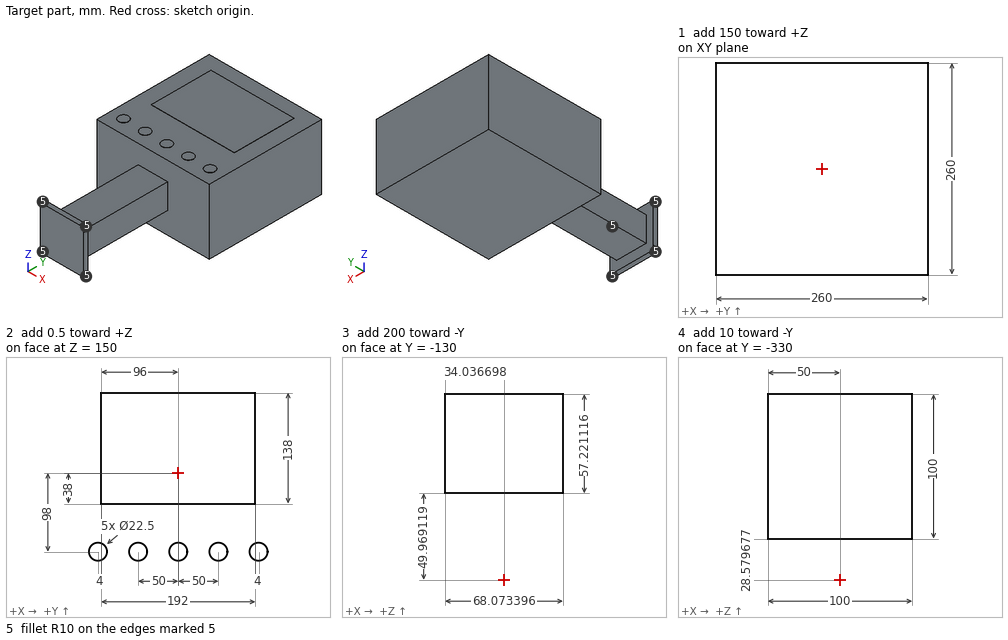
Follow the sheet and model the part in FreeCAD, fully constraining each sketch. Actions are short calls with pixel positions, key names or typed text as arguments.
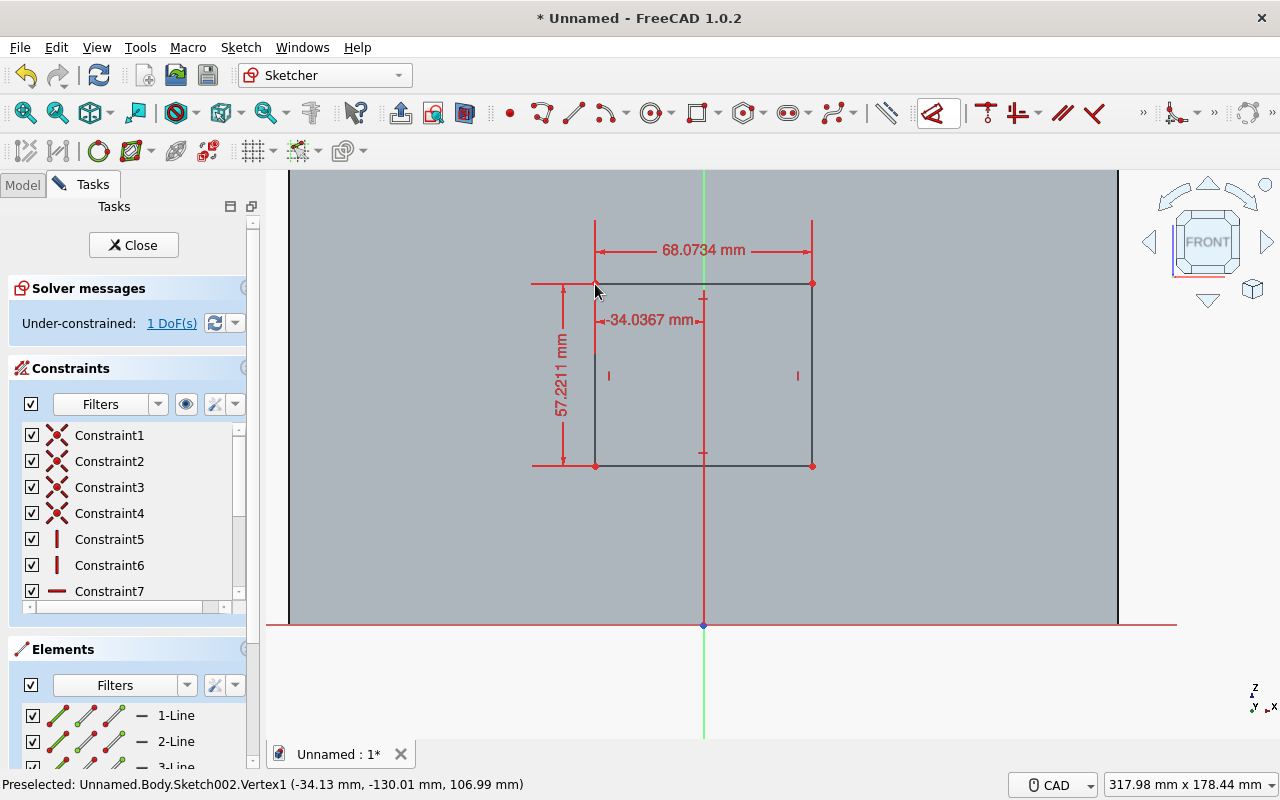
click(595, 466)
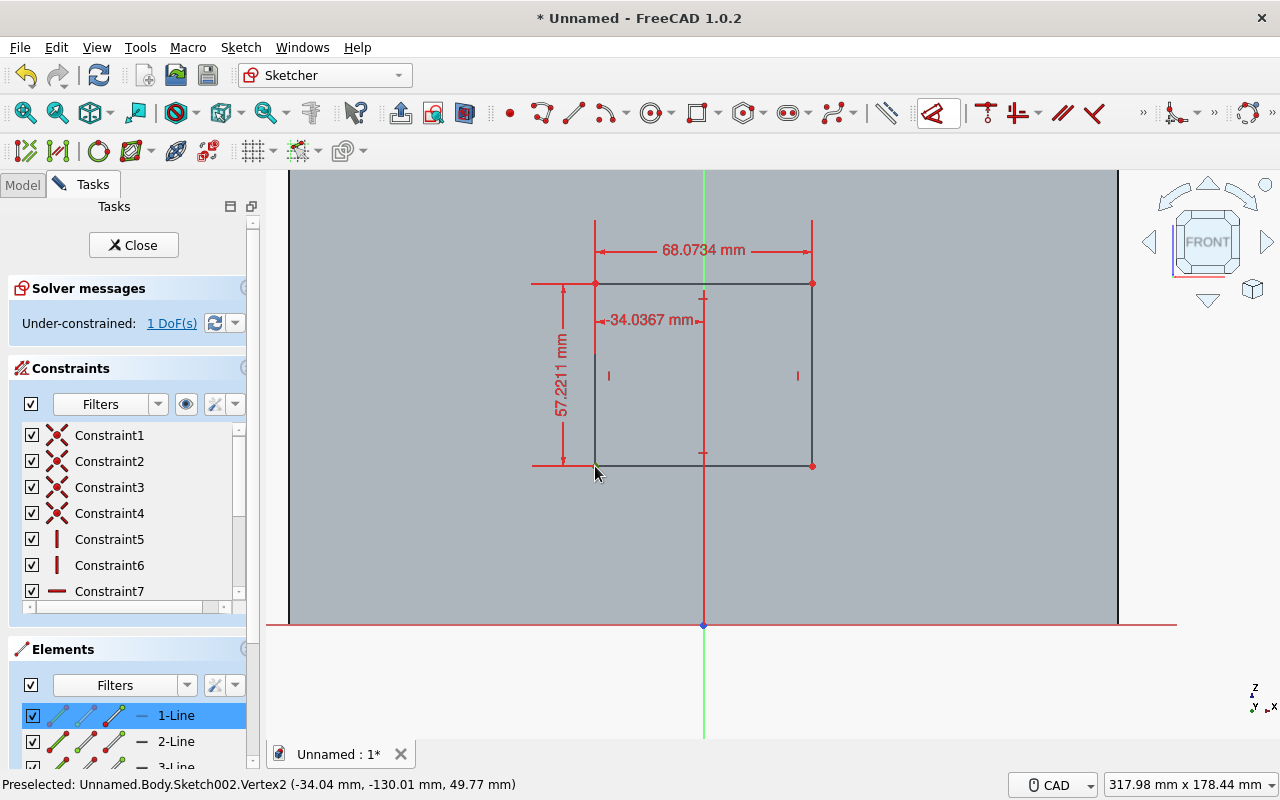
key(i)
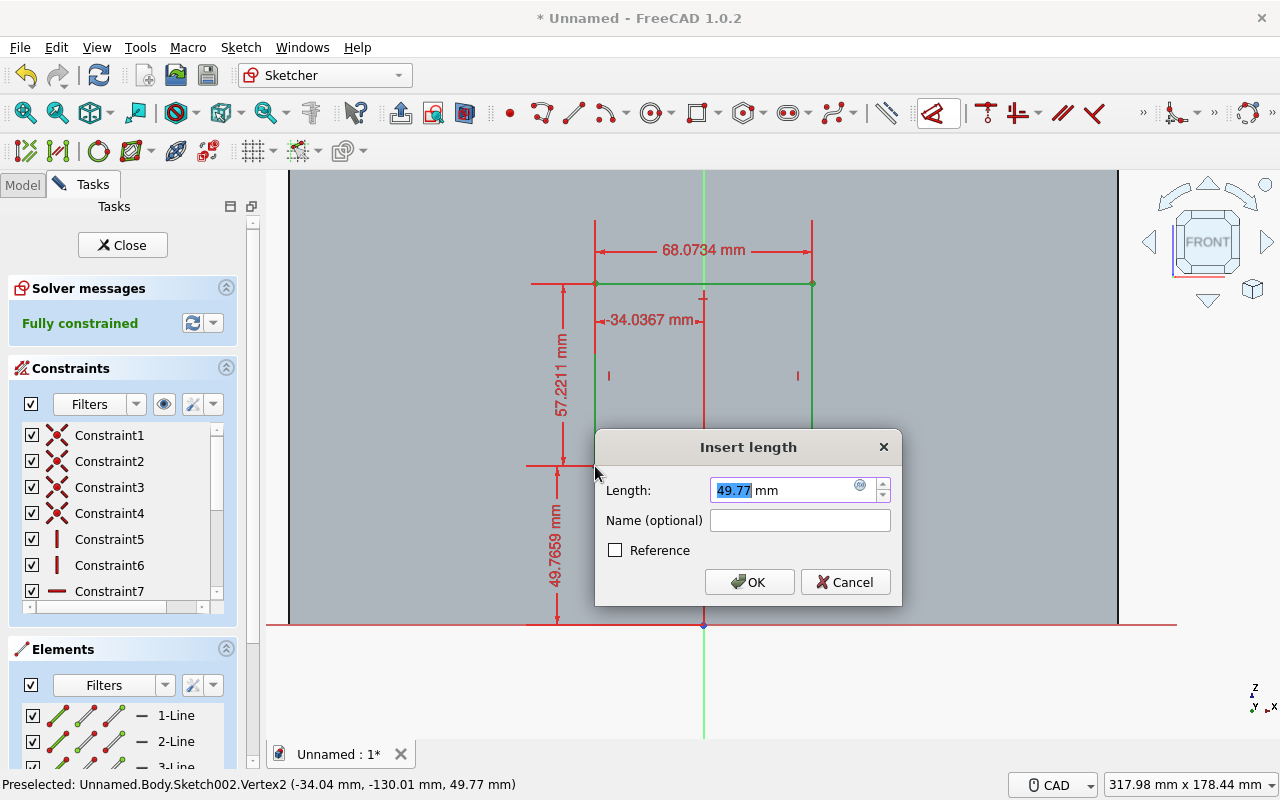
text(49.969119)
key(Return)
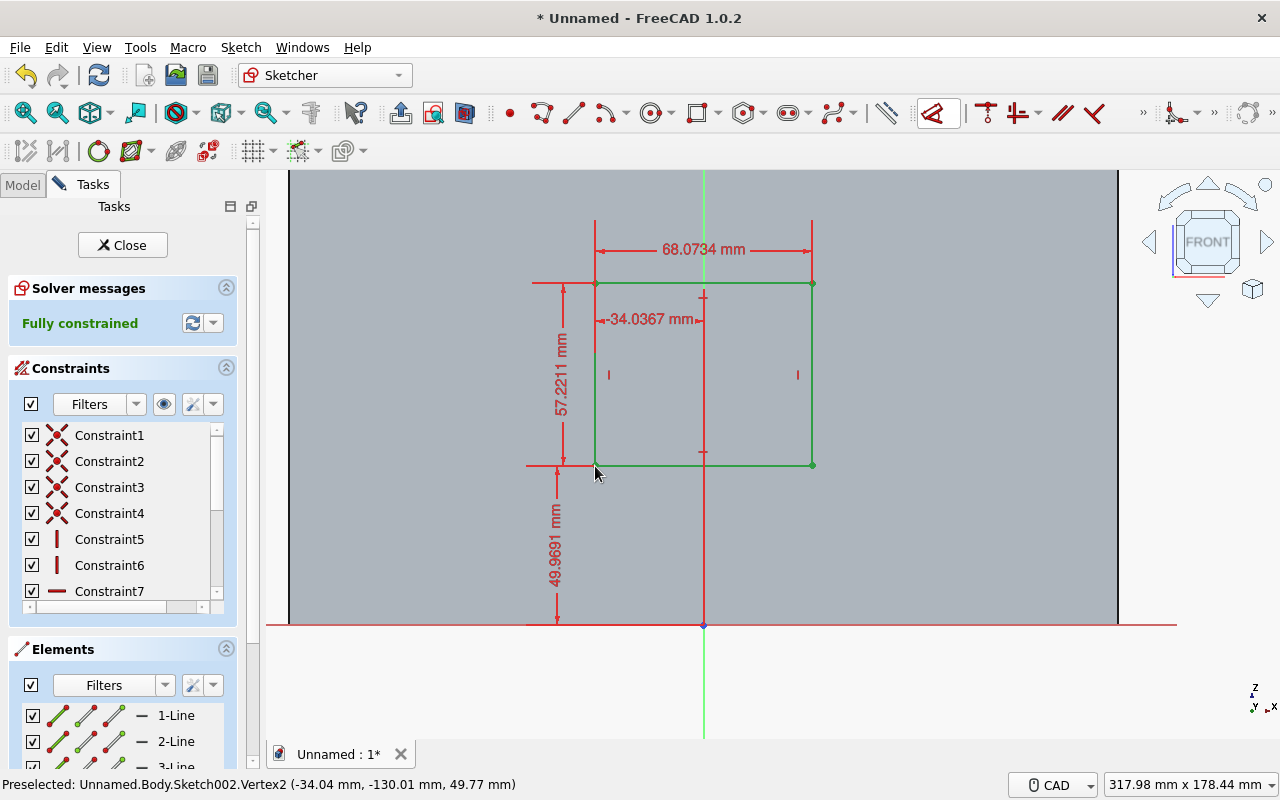
click(123, 245)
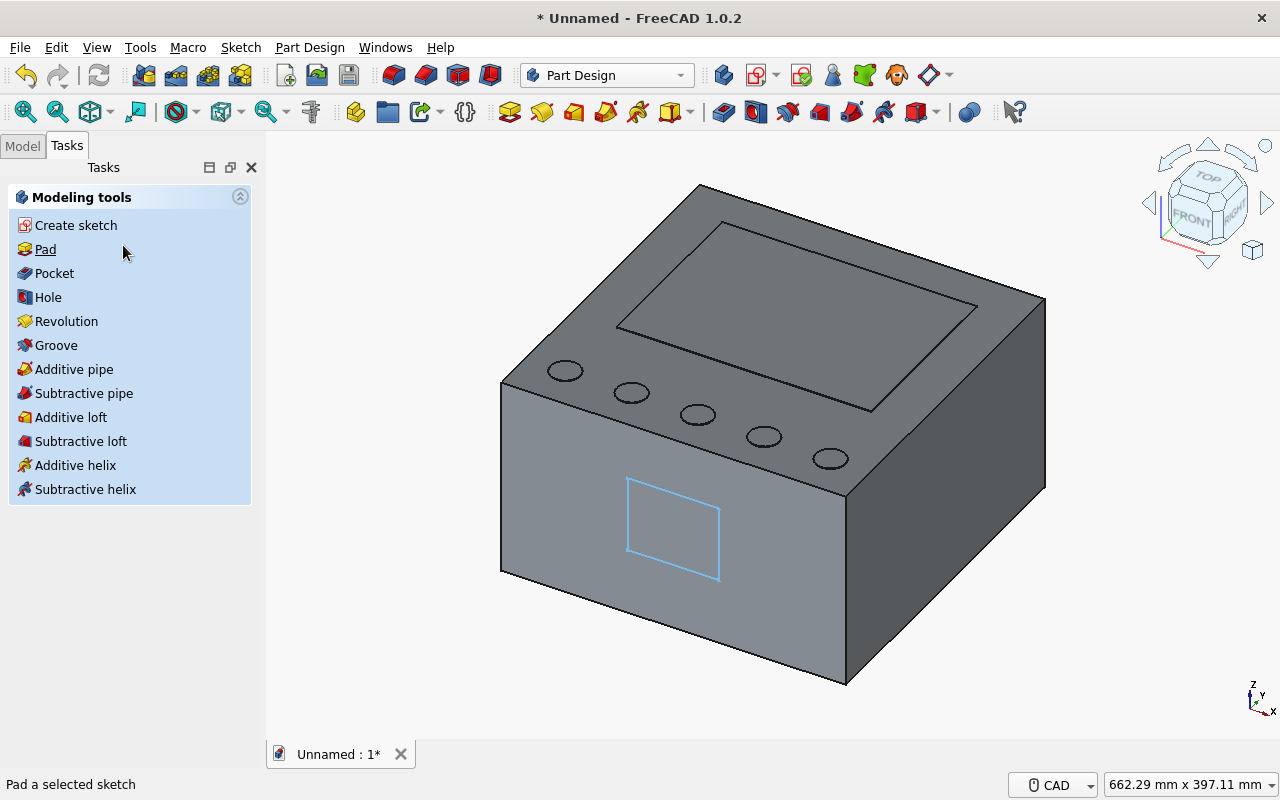
click(510, 112)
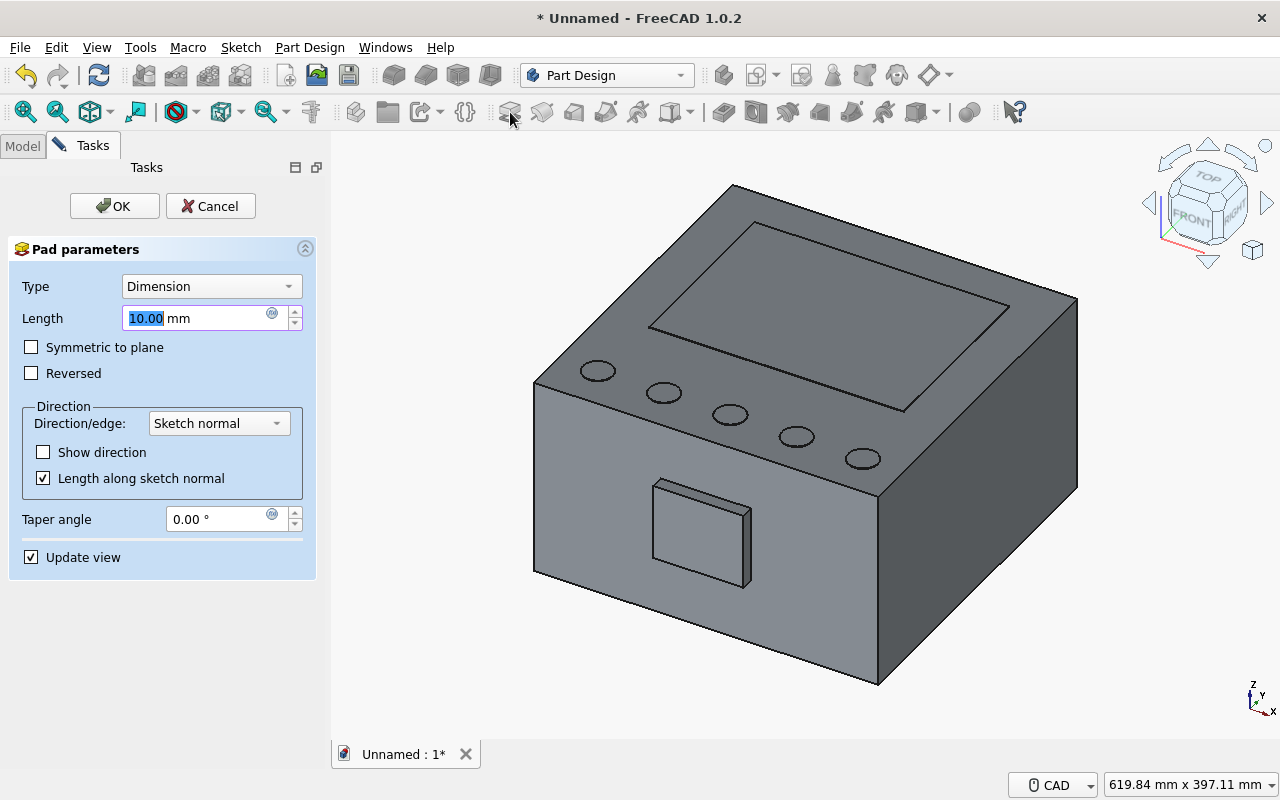
text(200)
key(Tab)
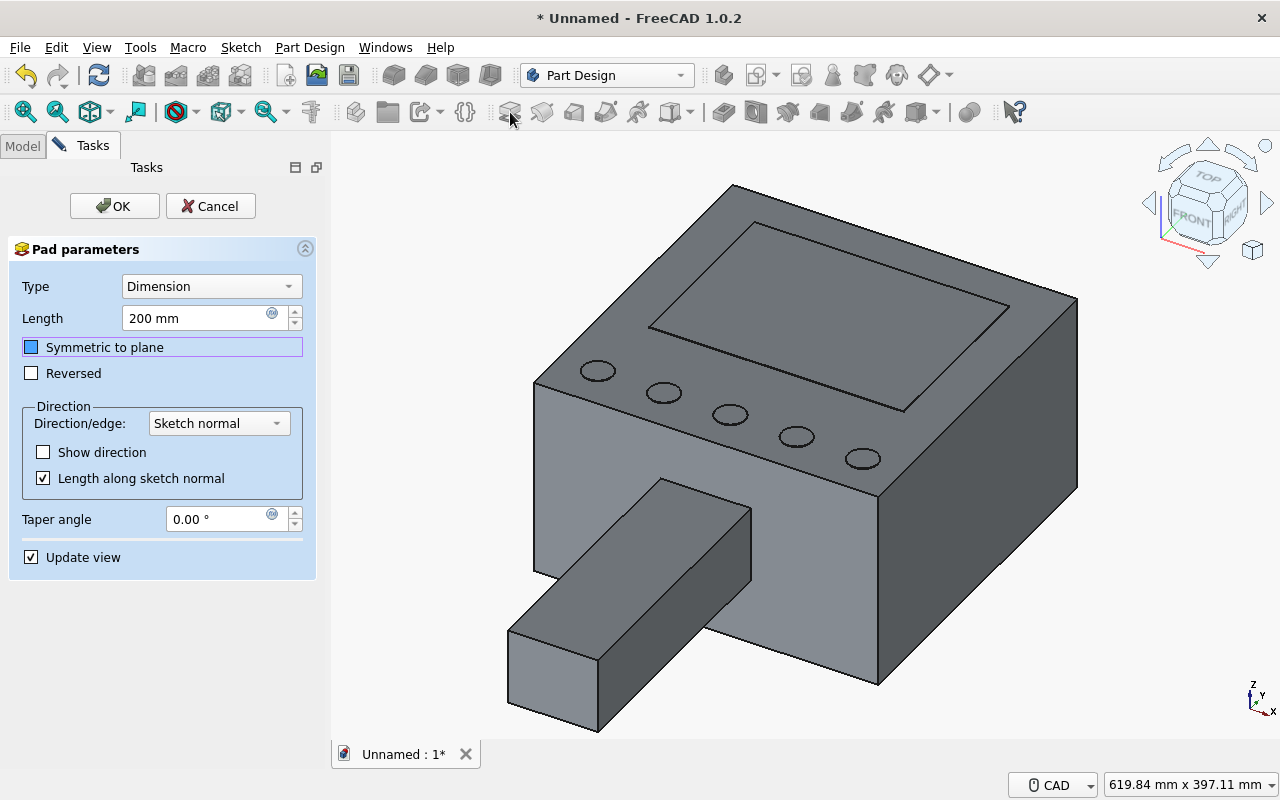
click(115, 206)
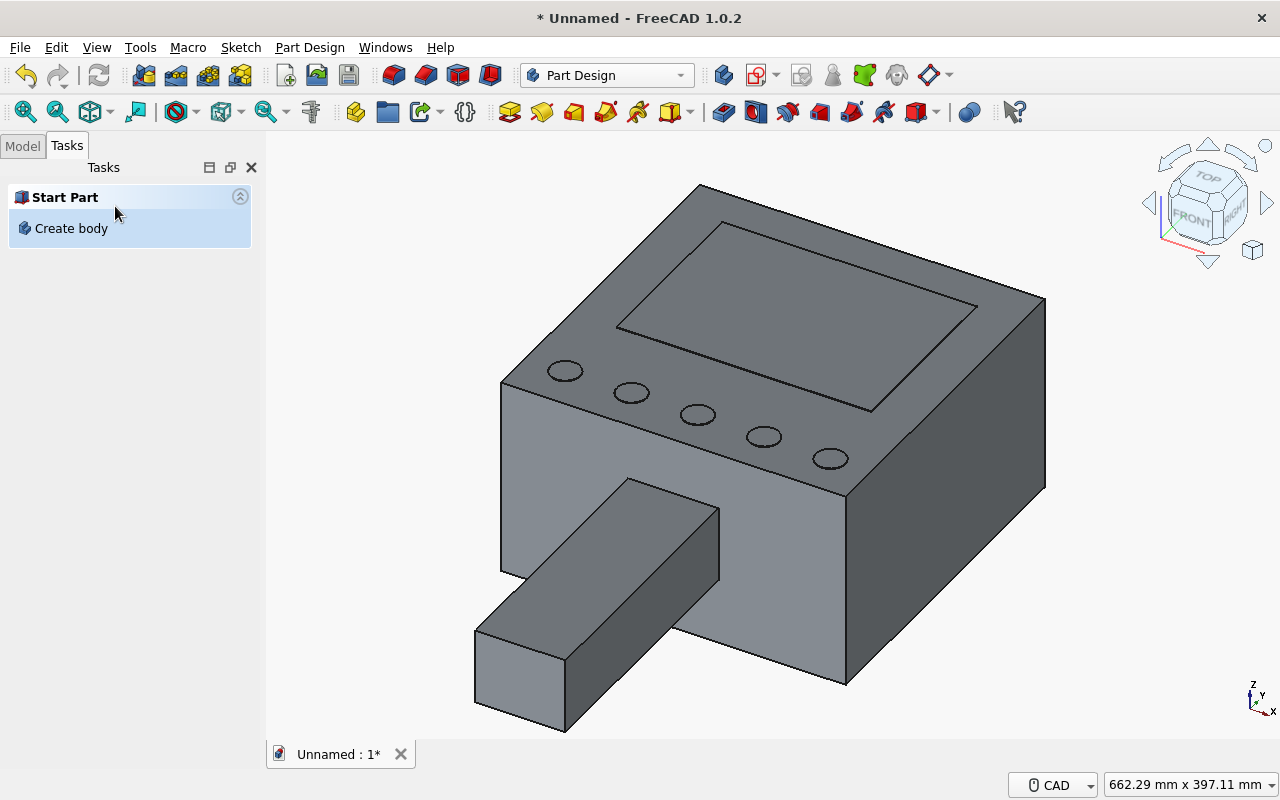
key(v)
key(f)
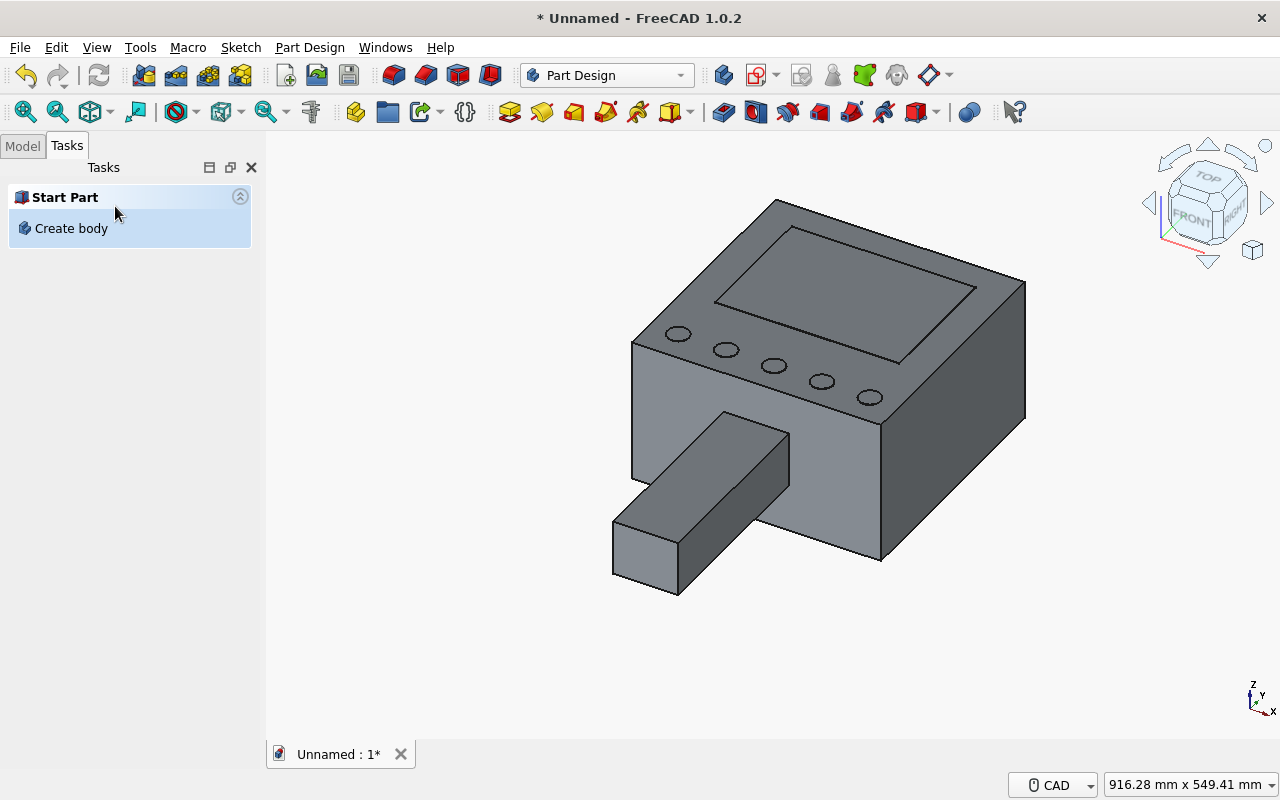
click(646, 557)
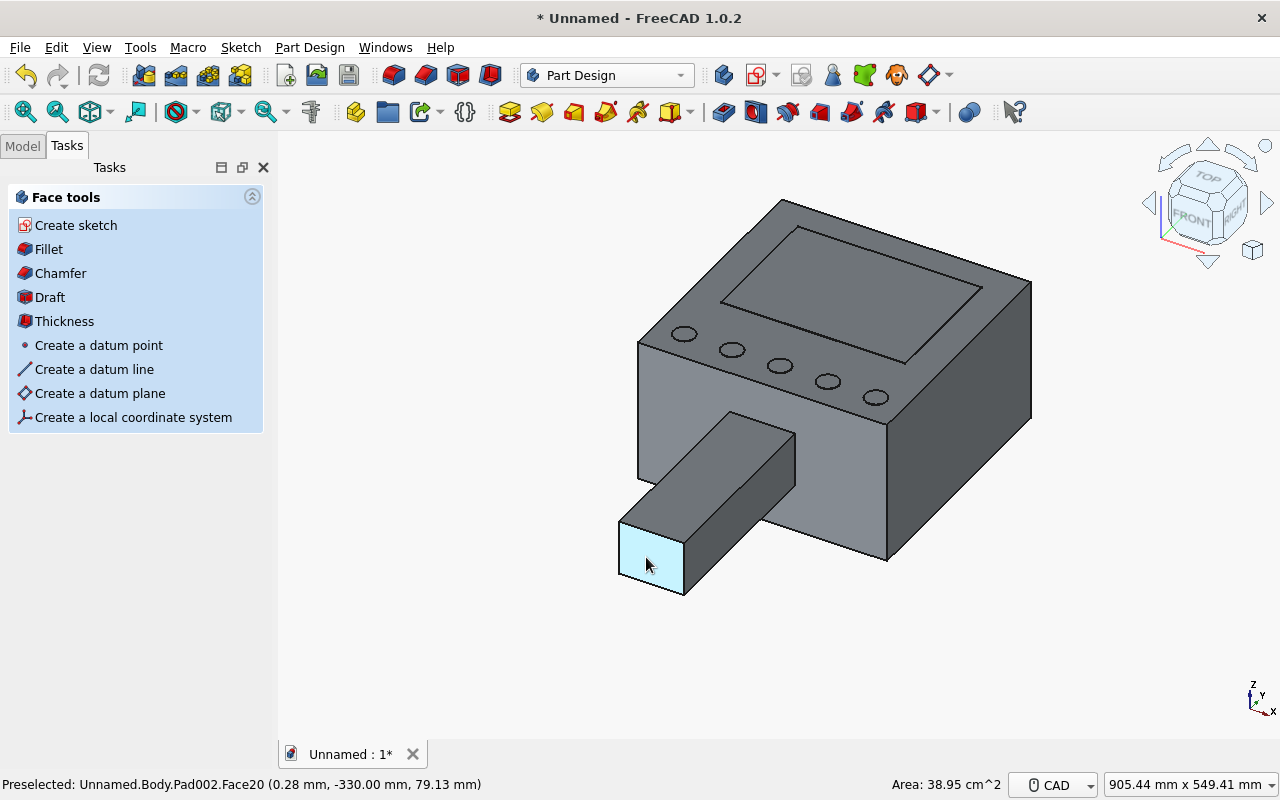
click(756, 76)